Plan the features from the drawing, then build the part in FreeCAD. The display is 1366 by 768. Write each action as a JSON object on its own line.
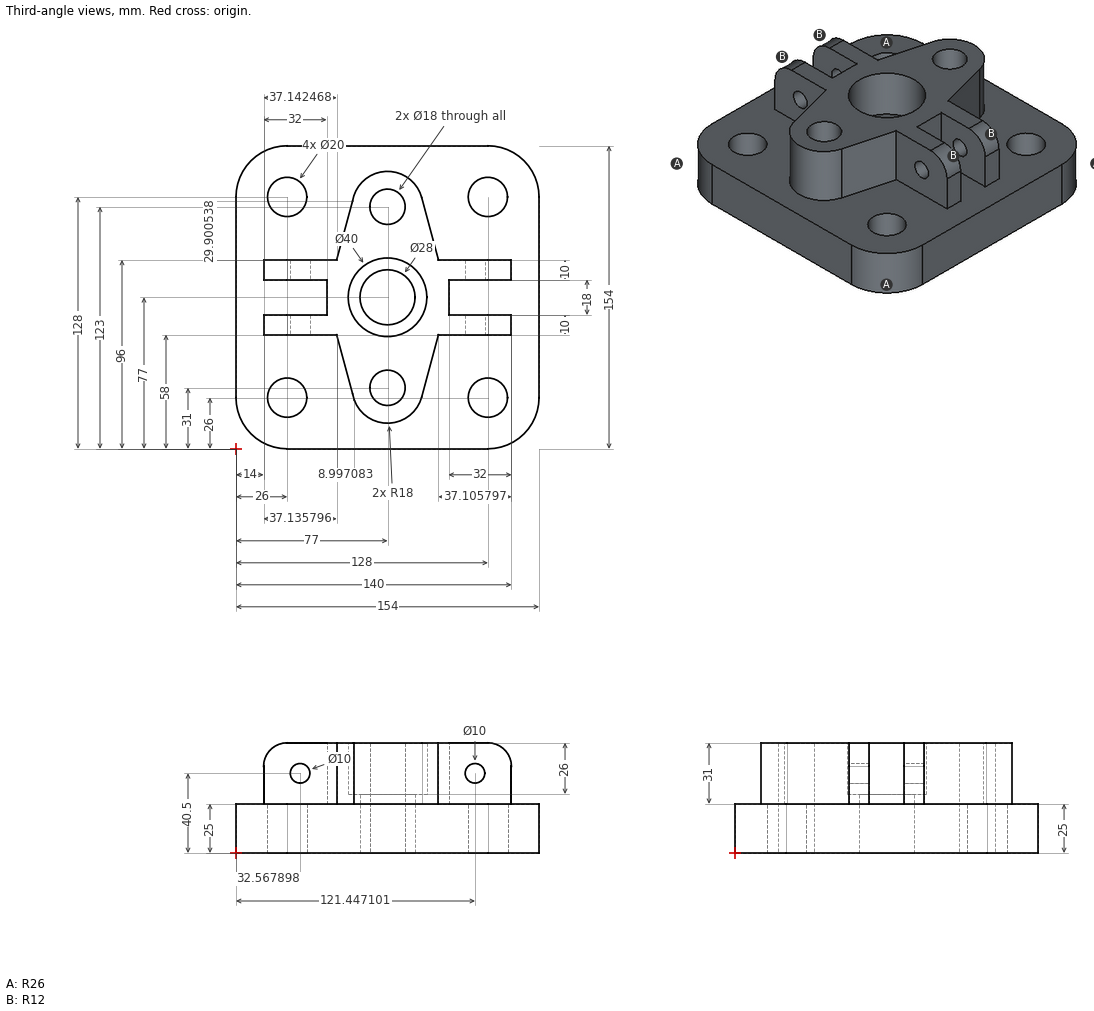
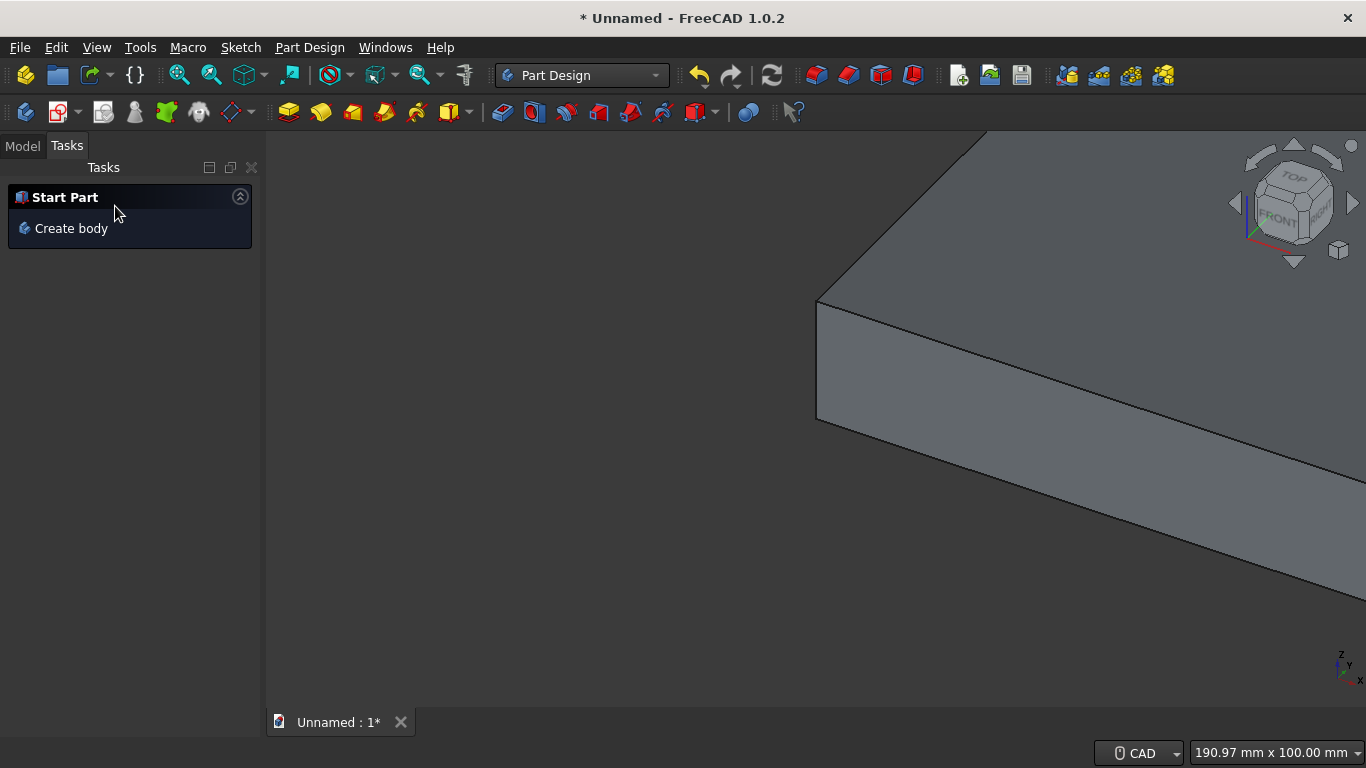
{"action": "left_click", "coordinate": [180, 76]}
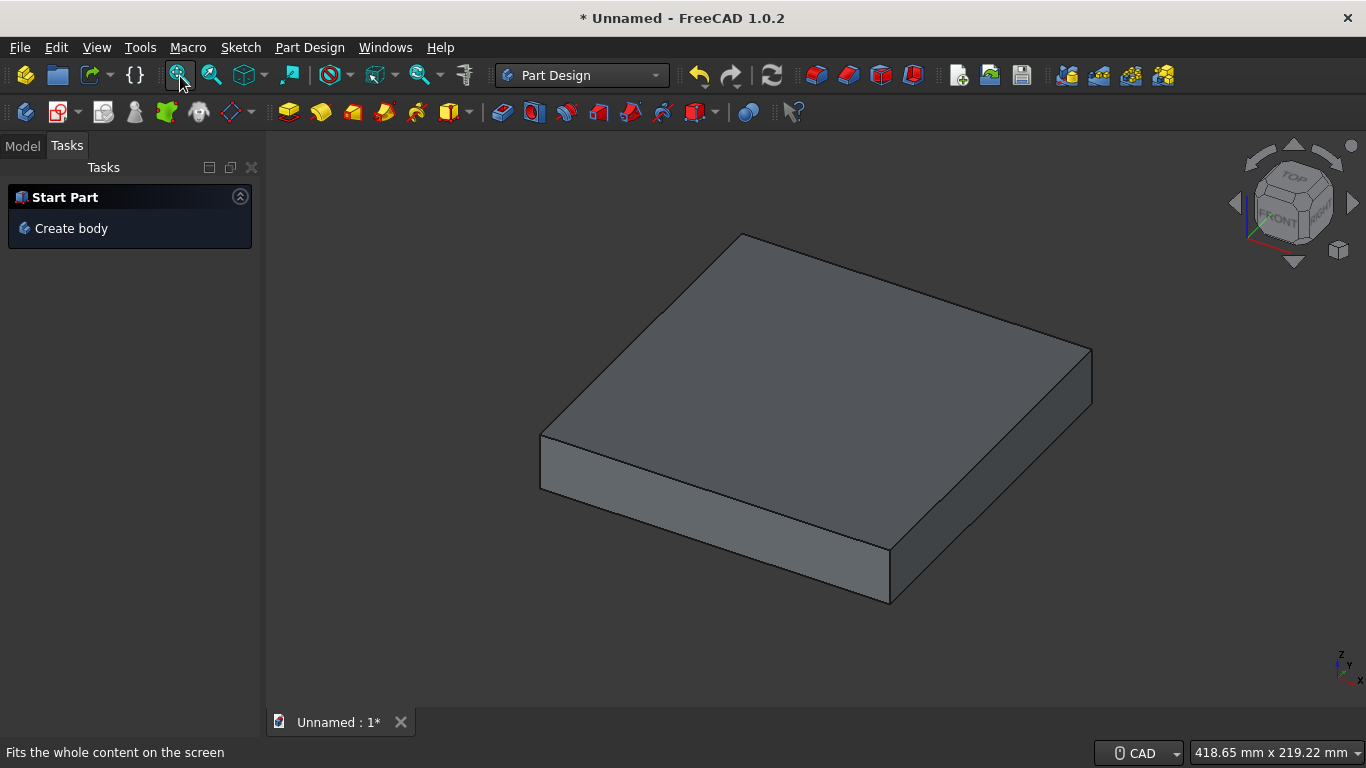
{"action": "left_click", "coordinate": [890, 577]}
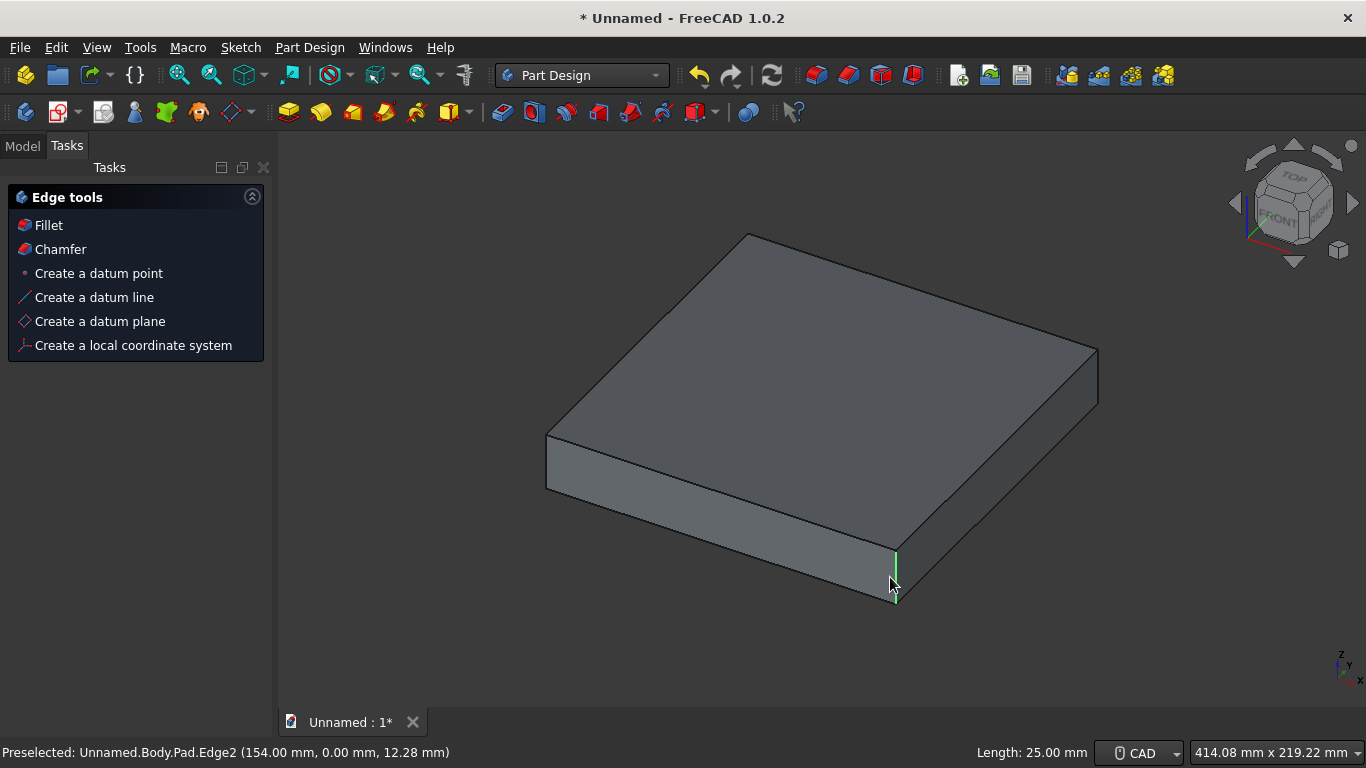
{"action": "key", "text": "0"}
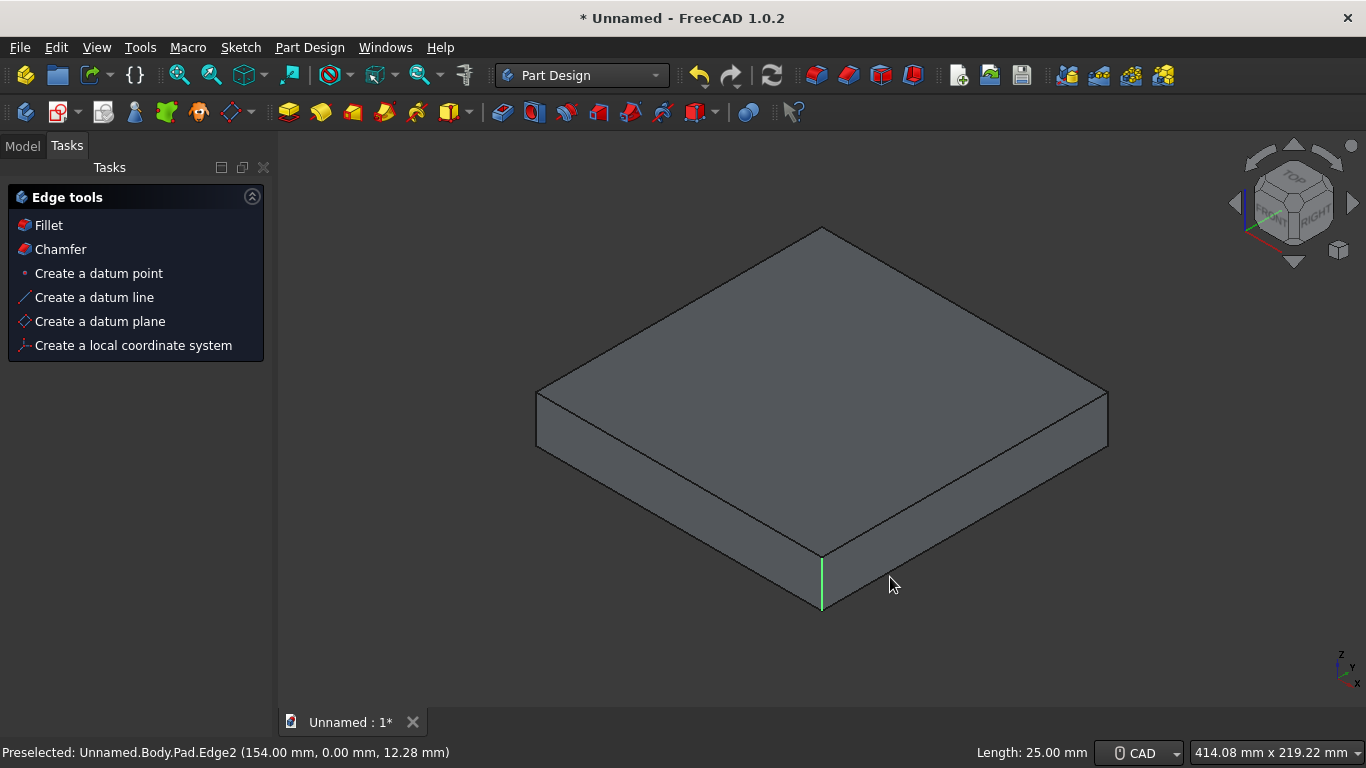
{"action": "key", "text": "2"}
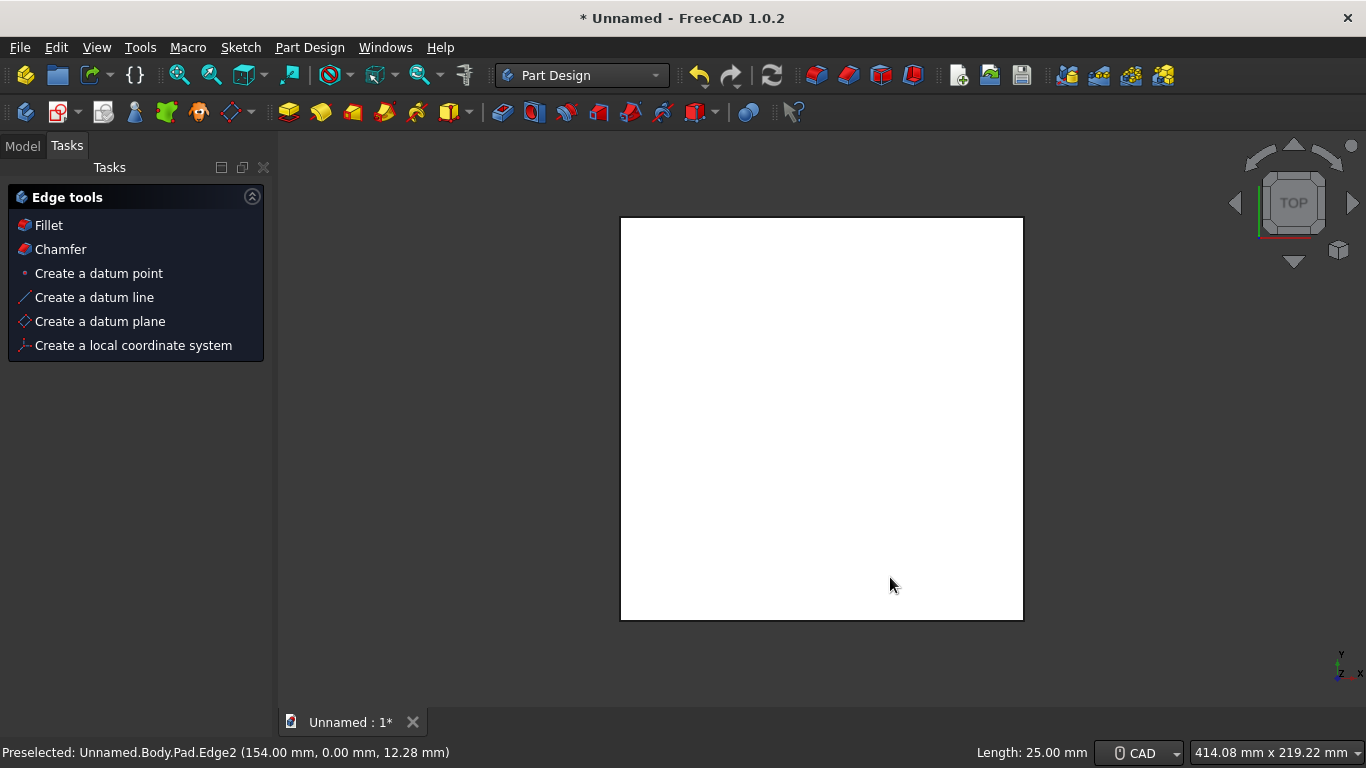
{"action": "key", "text": "1"}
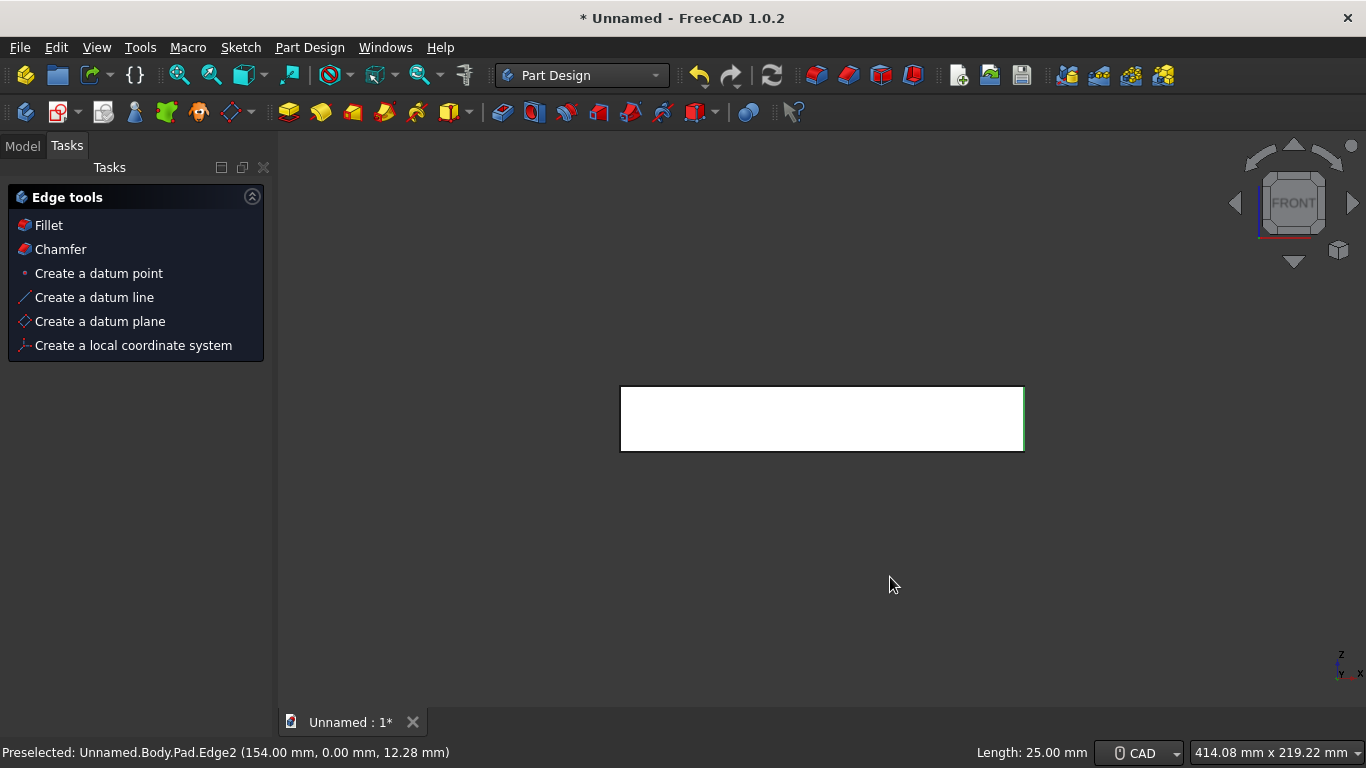
{"action": "left_click", "coordinate": [180, 76]}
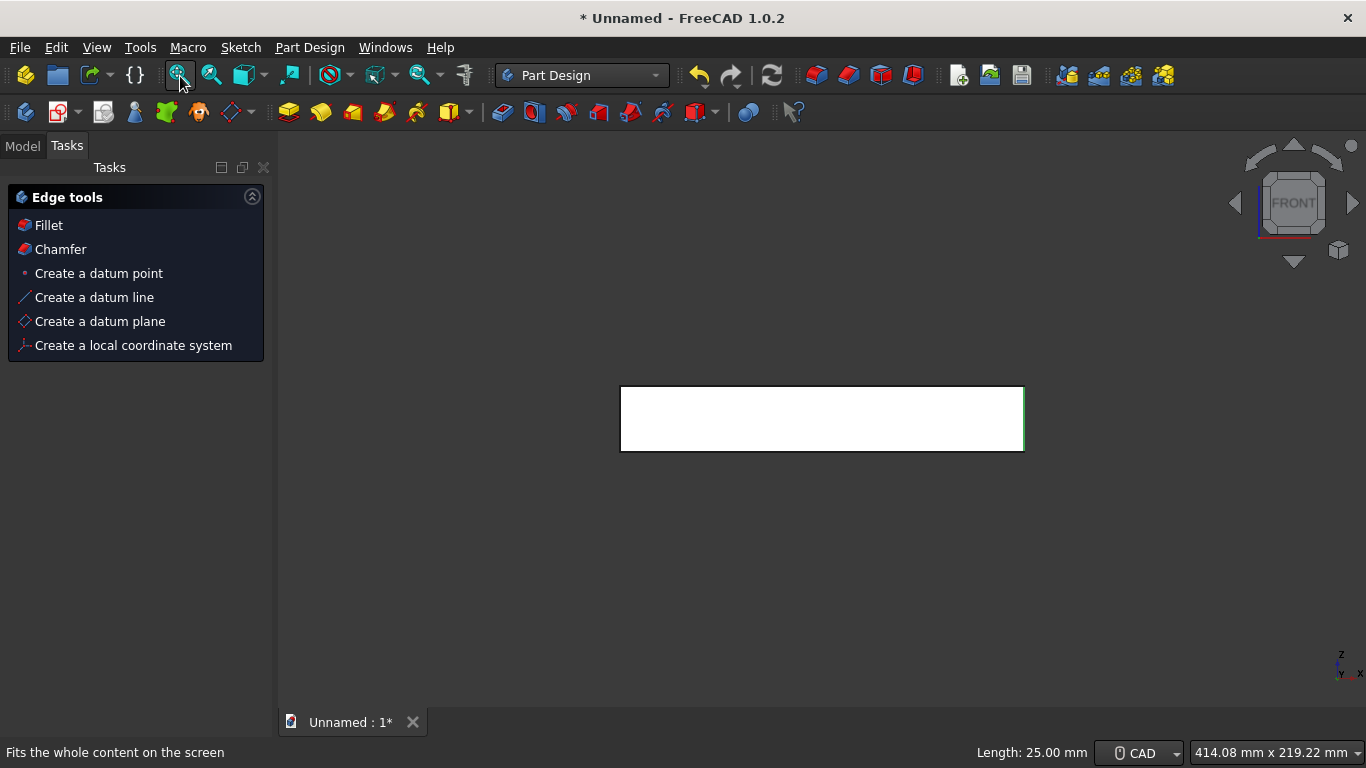
{"action": "left_click", "coordinate": [620, 418], "text": "ctrl"}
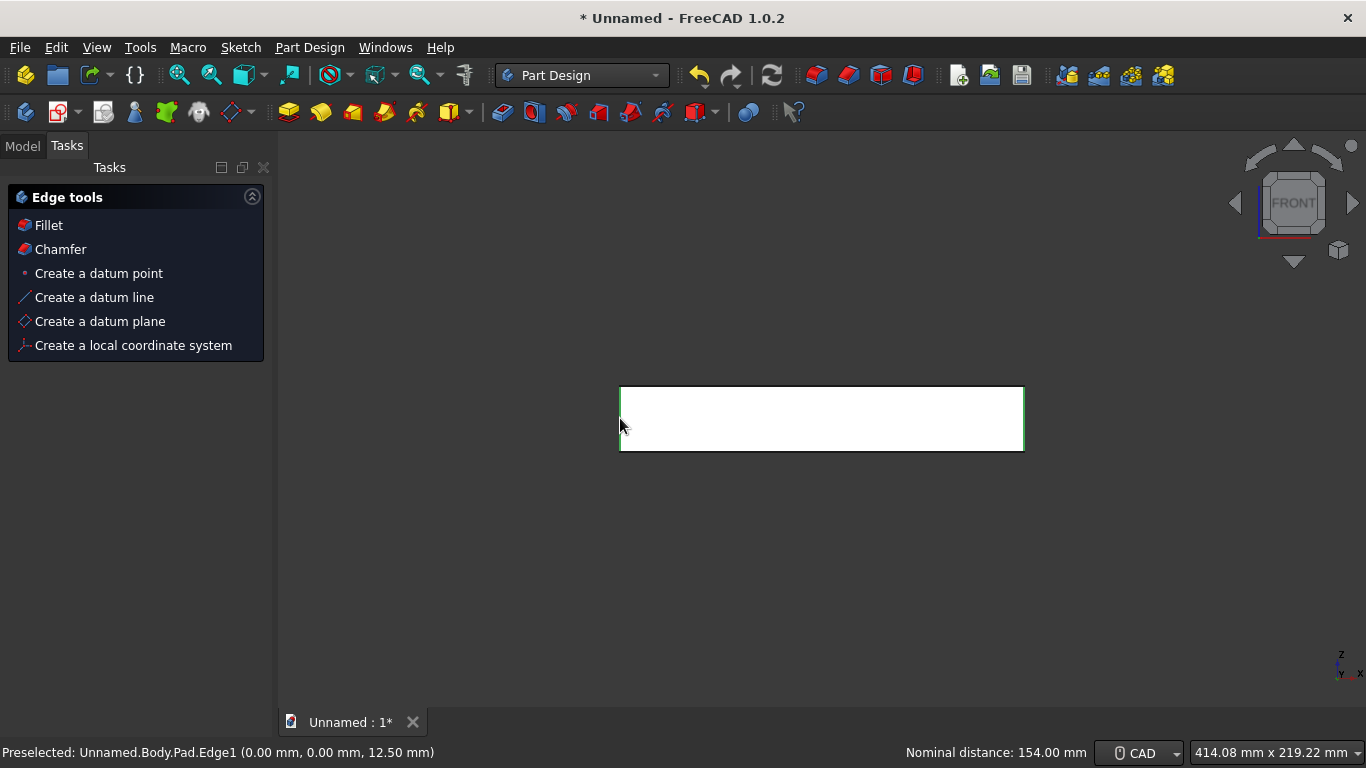
{"action": "key", "text": "3"}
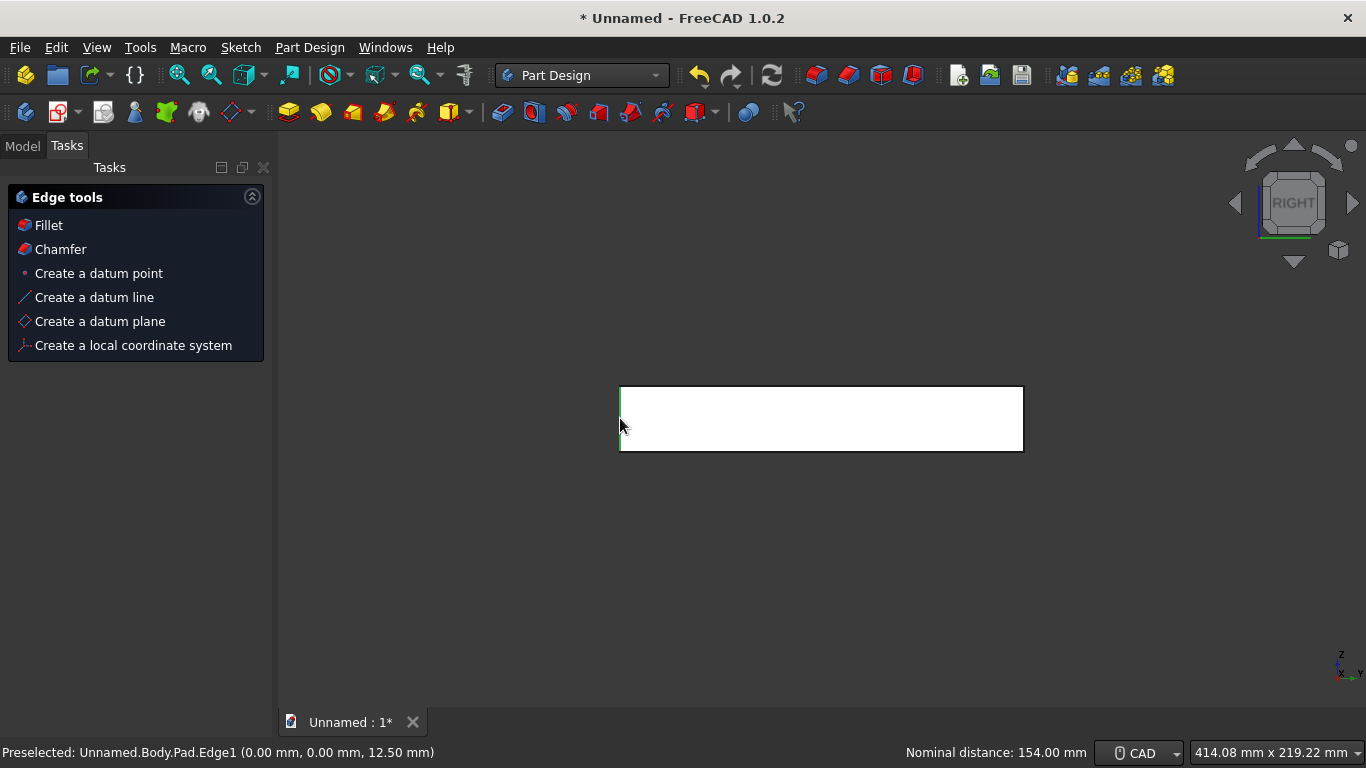
{"action": "left_click", "coordinate": [180, 76]}